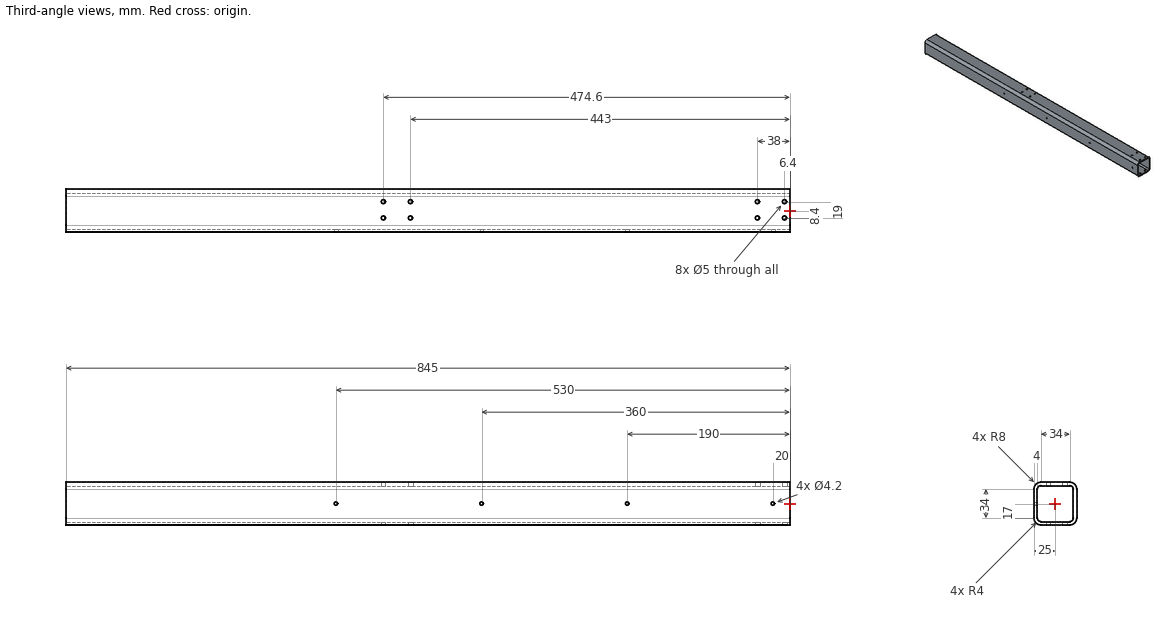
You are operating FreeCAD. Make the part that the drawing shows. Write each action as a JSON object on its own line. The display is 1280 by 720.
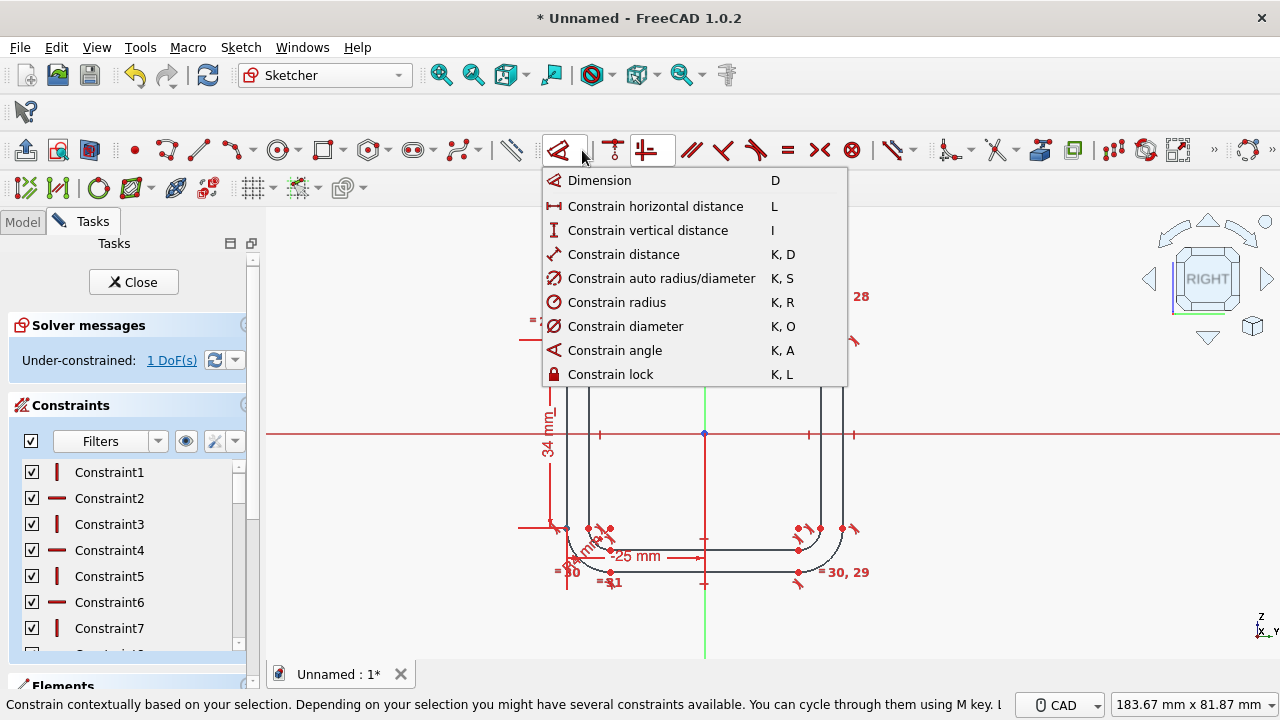
{"action": "left_click", "coordinate": [695, 230]}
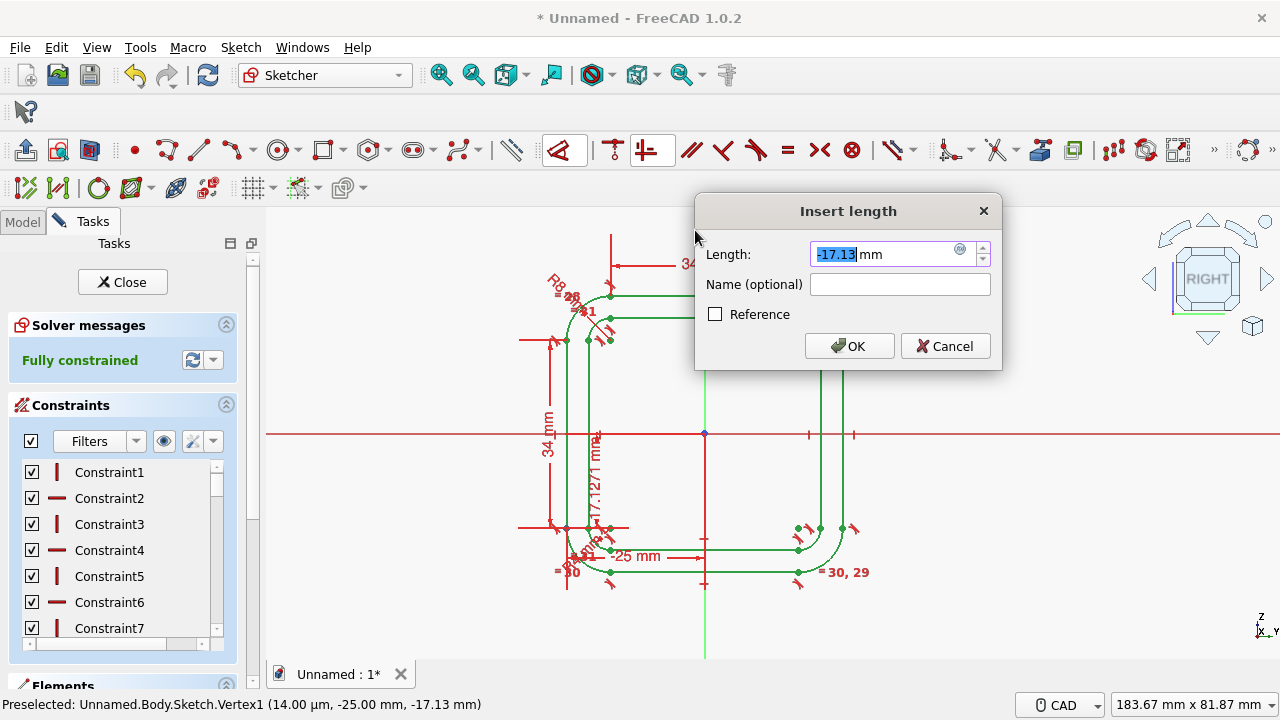
{"action": "type", "text": "-17"}
{"action": "key", "text": "Return"}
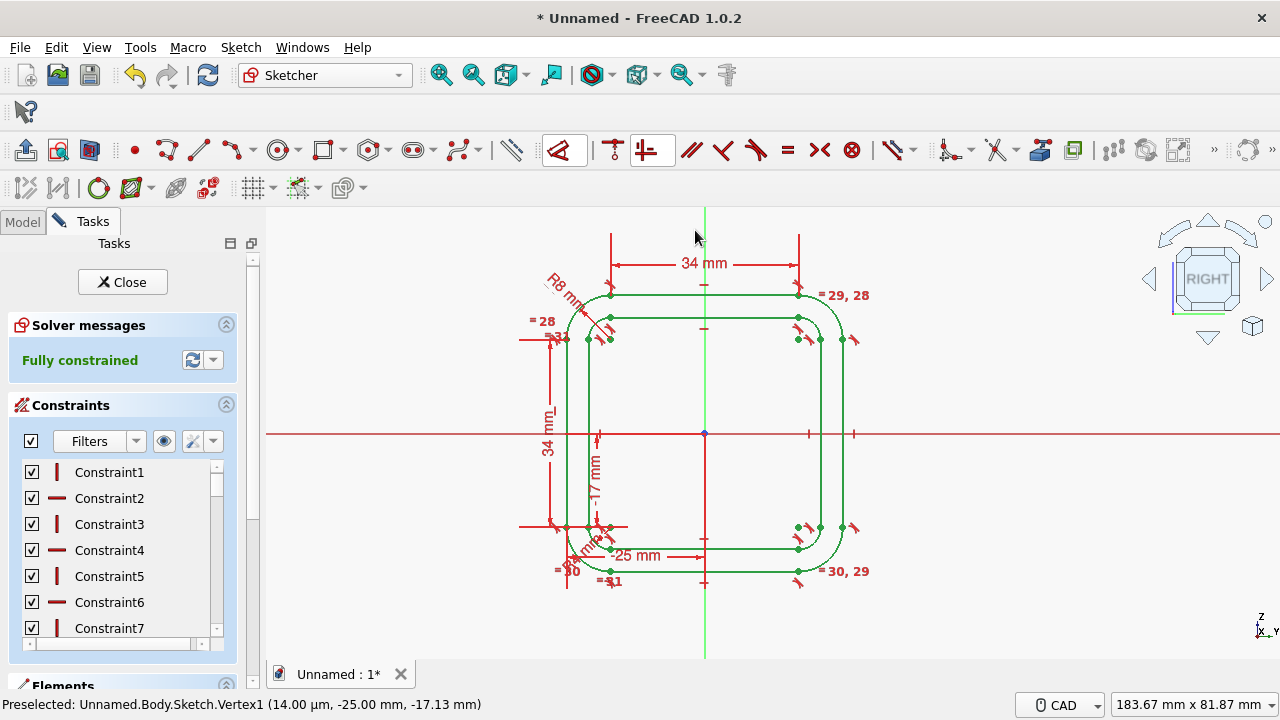
{"action": "left_click", "coordinate": [123, 282]}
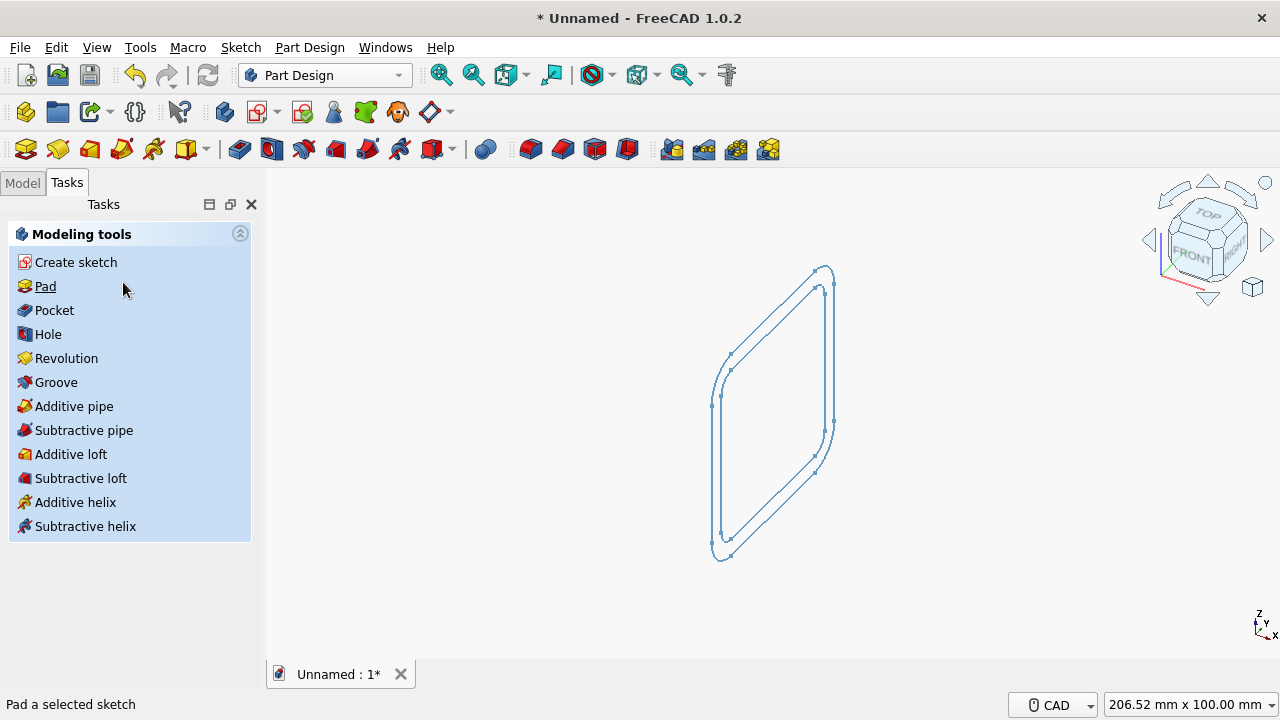
{"action": "left_click", "coordinate": [26, 150]}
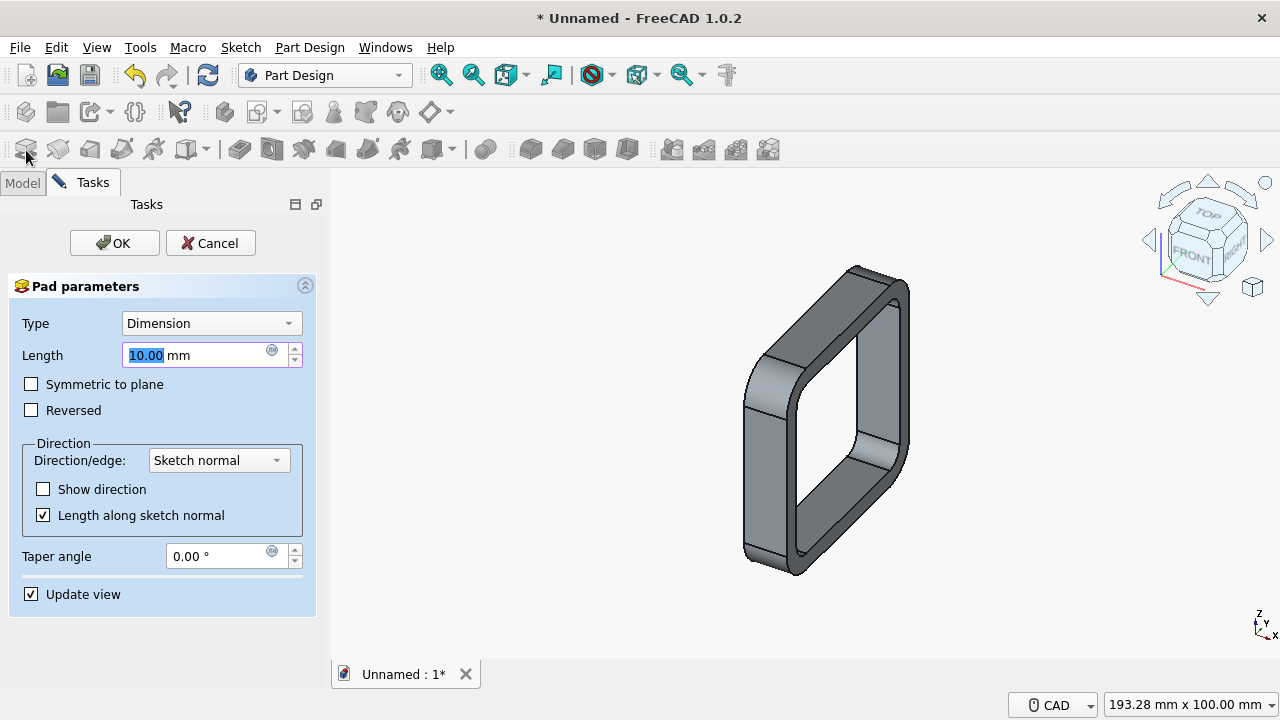
{"action": "type", "text": "845"}
{"action": "key", "text": "Tab"}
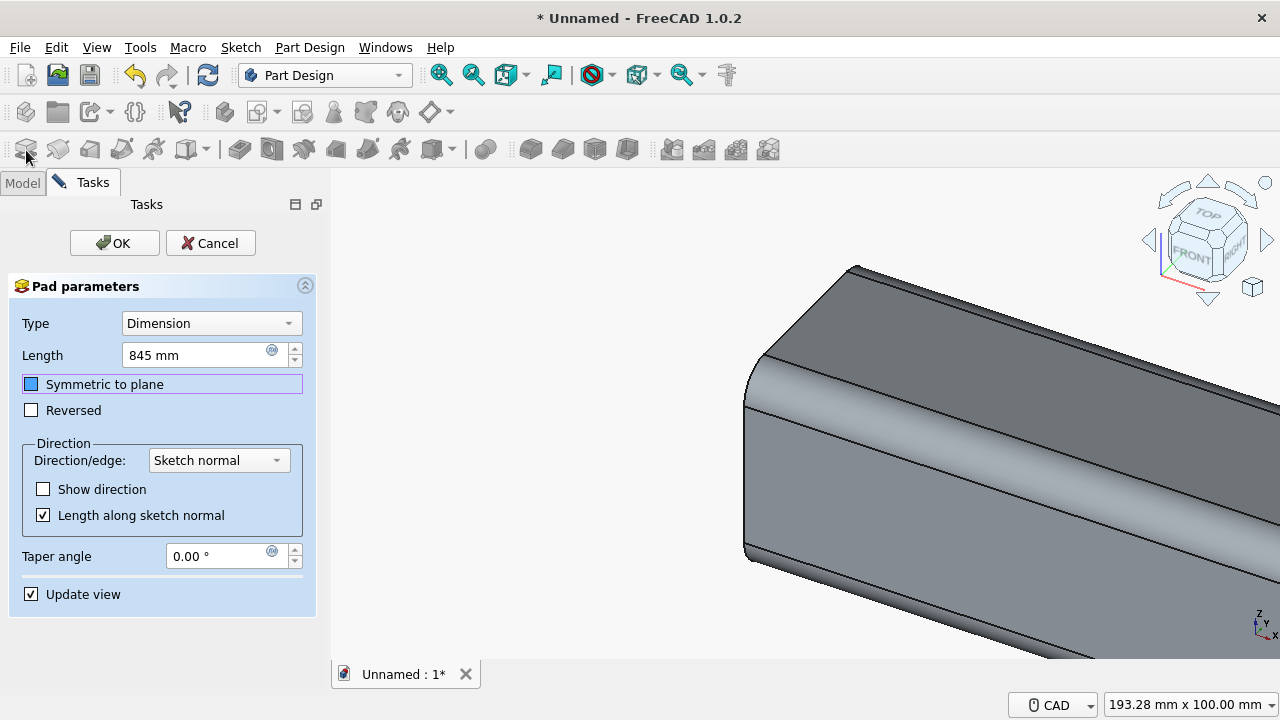
{"action": "left_click", "coordinate": [30, 410]}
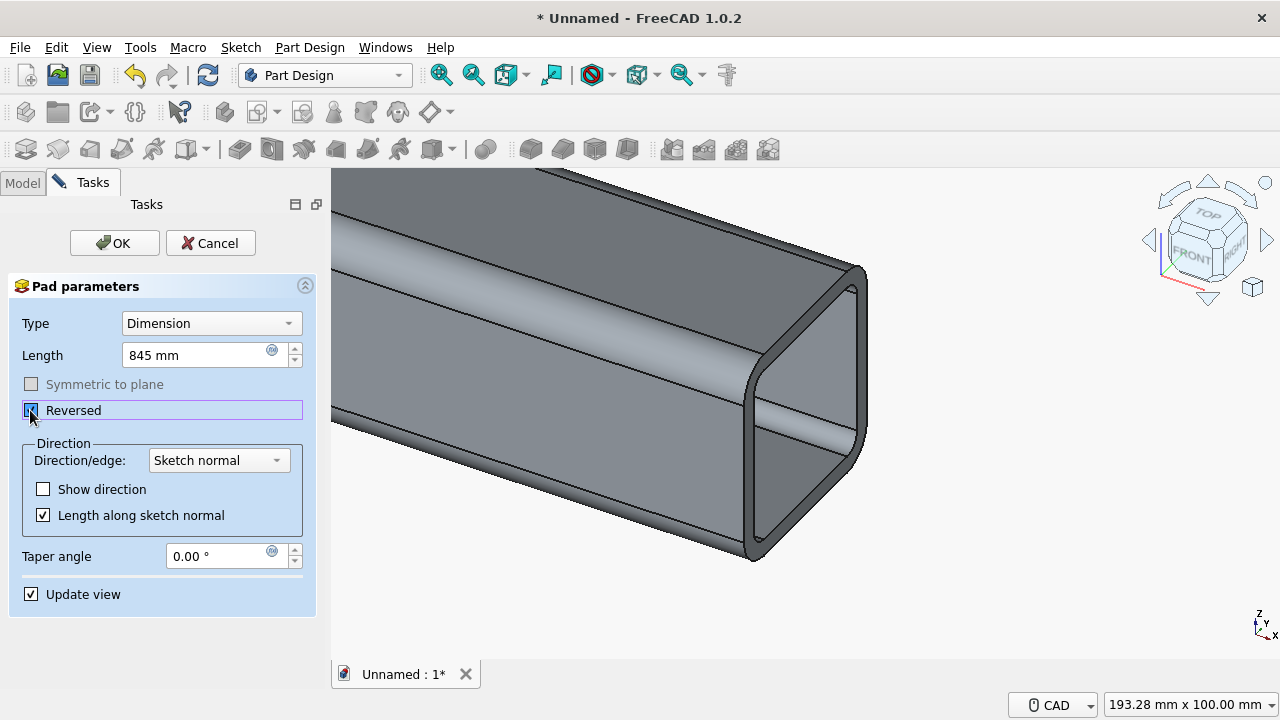
{"action": "left_click", "coordinate": [115, 243]}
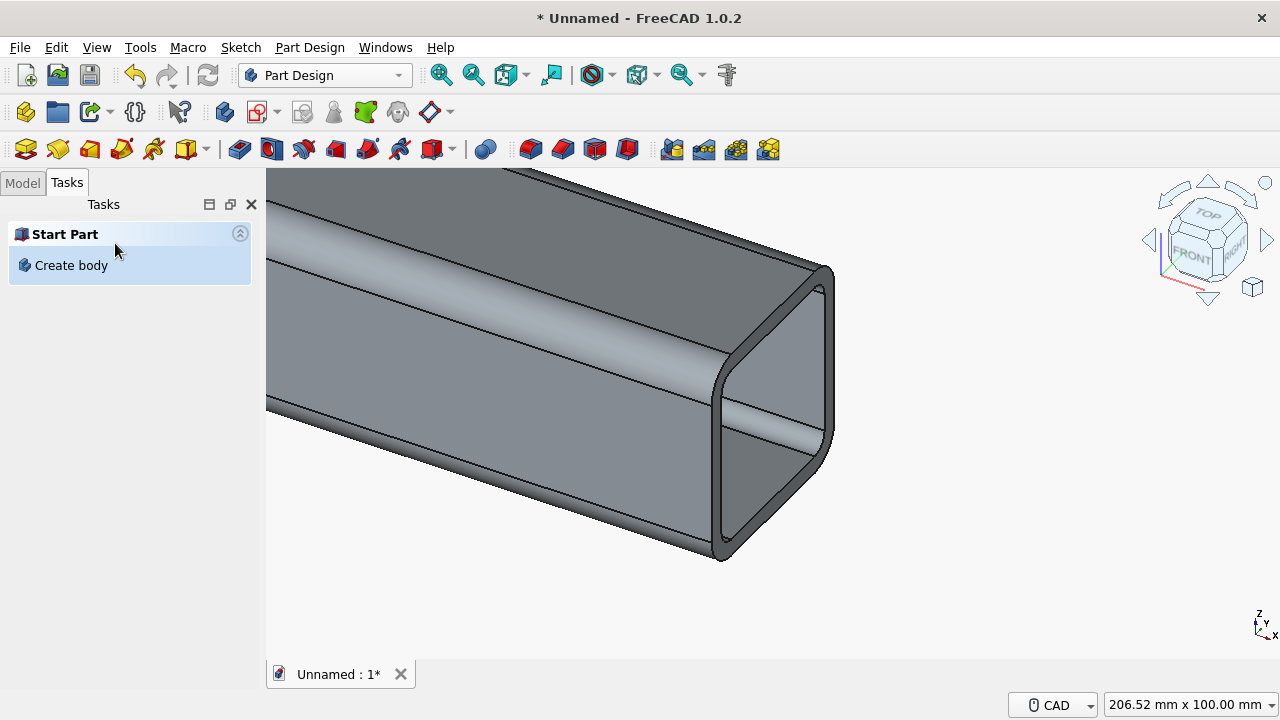
{"action": "left_click", "coordinate": [442, 76]}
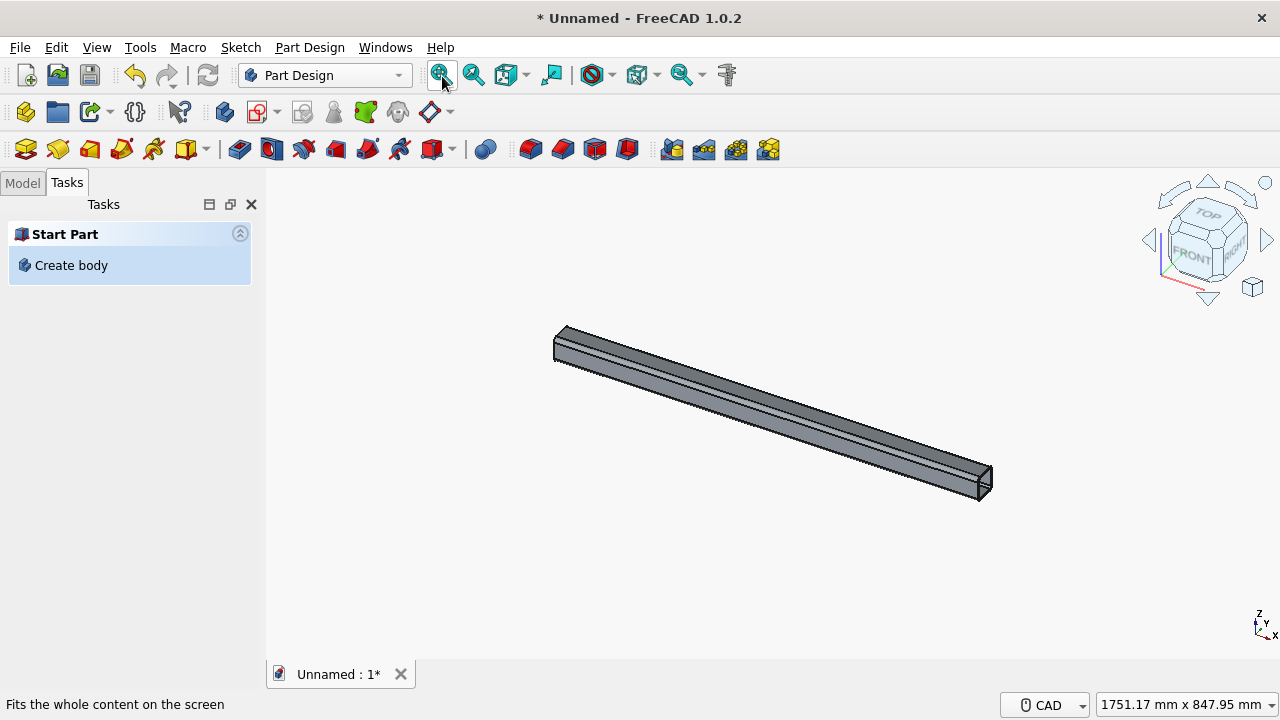
{"action": "key", "text": "5"}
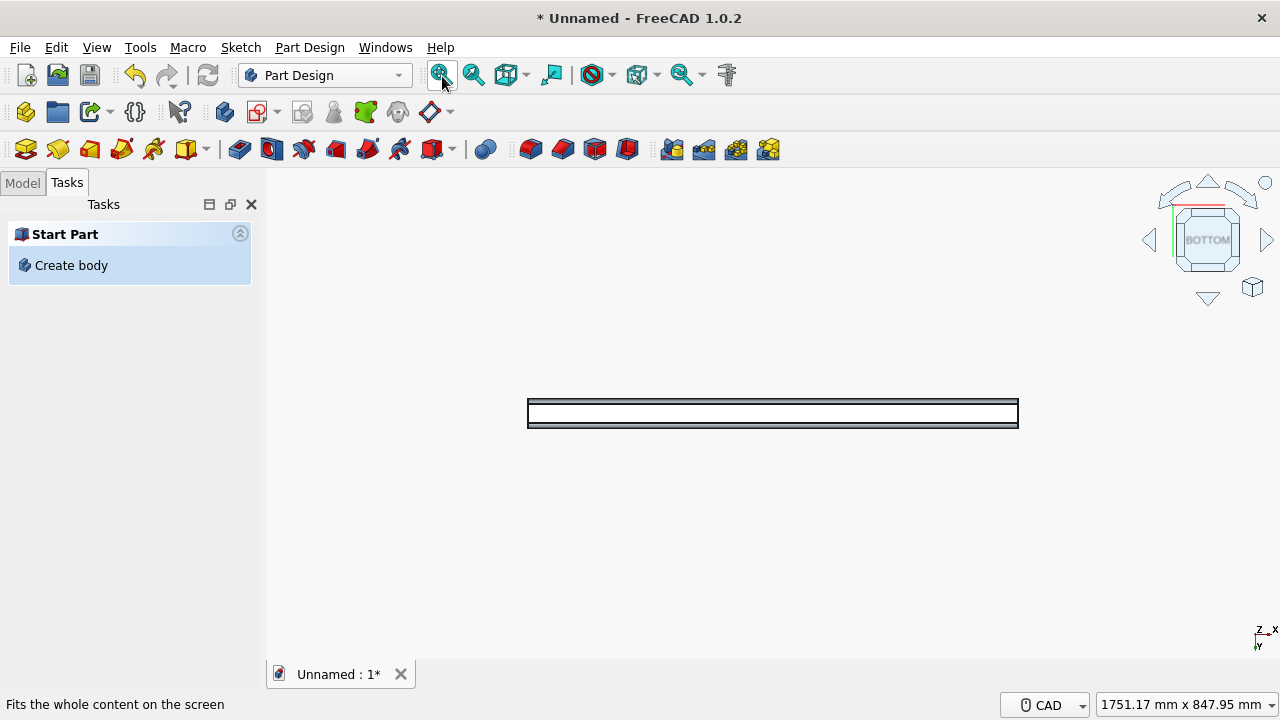
{"action": "left_click", "coordinate": [773, 412]}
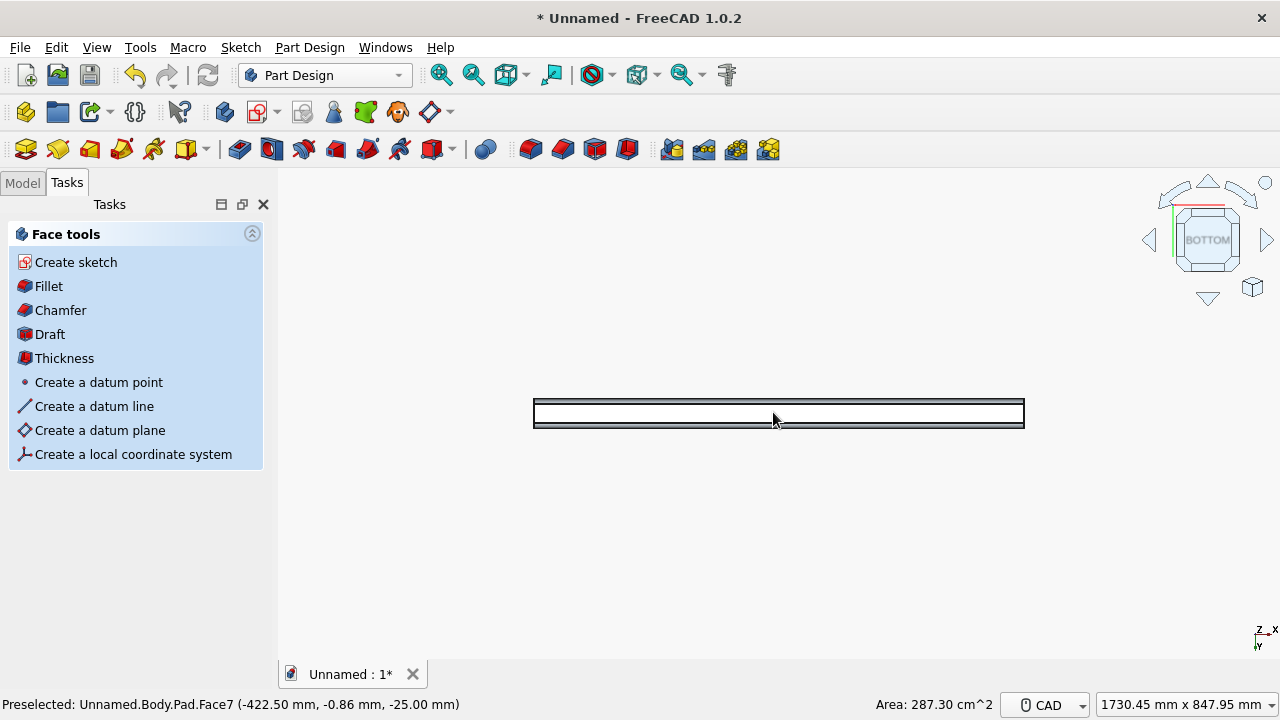
{"action": "left_click", "coordinate": [258, 112]}